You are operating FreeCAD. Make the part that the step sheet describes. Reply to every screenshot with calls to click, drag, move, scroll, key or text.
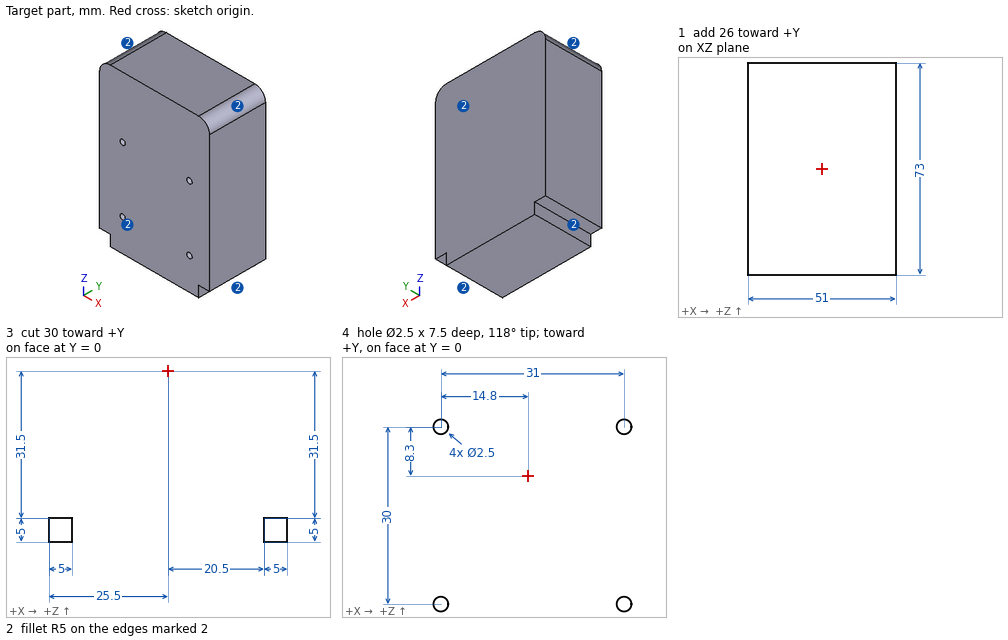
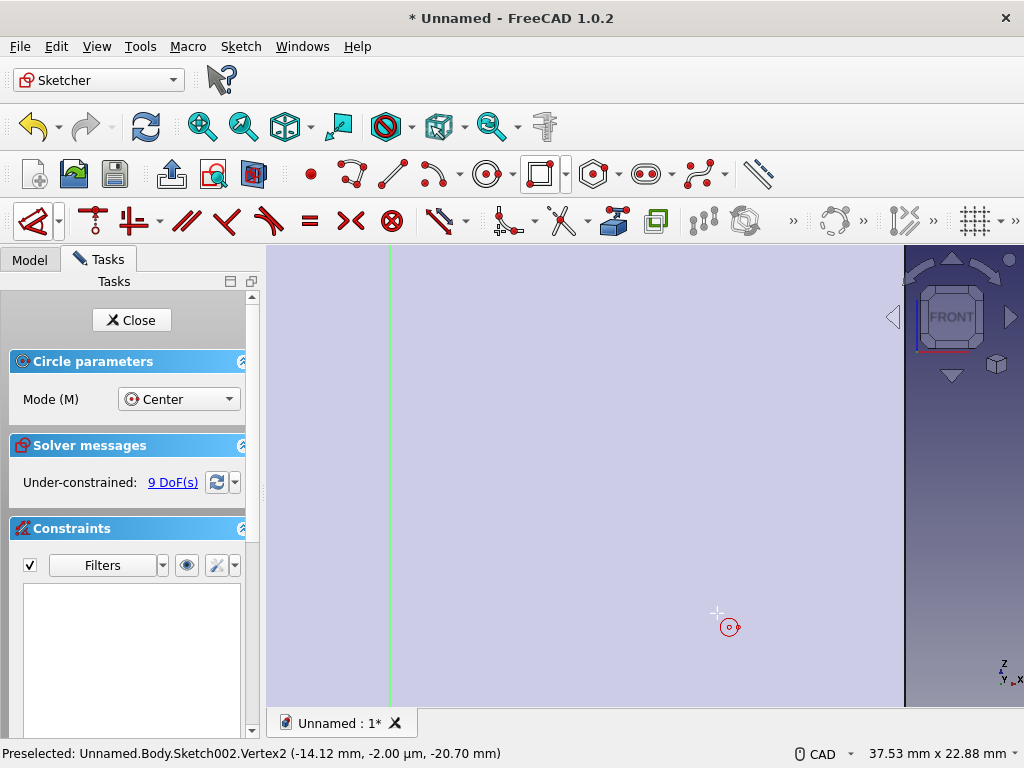
click(717, 611)
click(735, 593)
key(Escape)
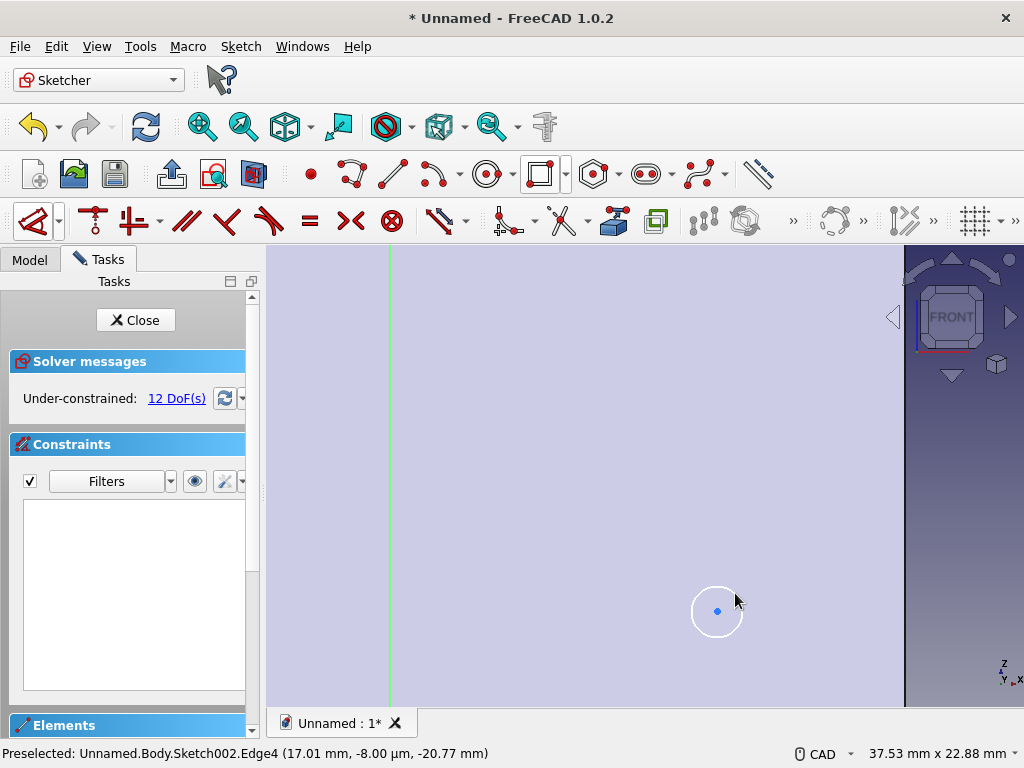
scroll(717, 613, down, 4)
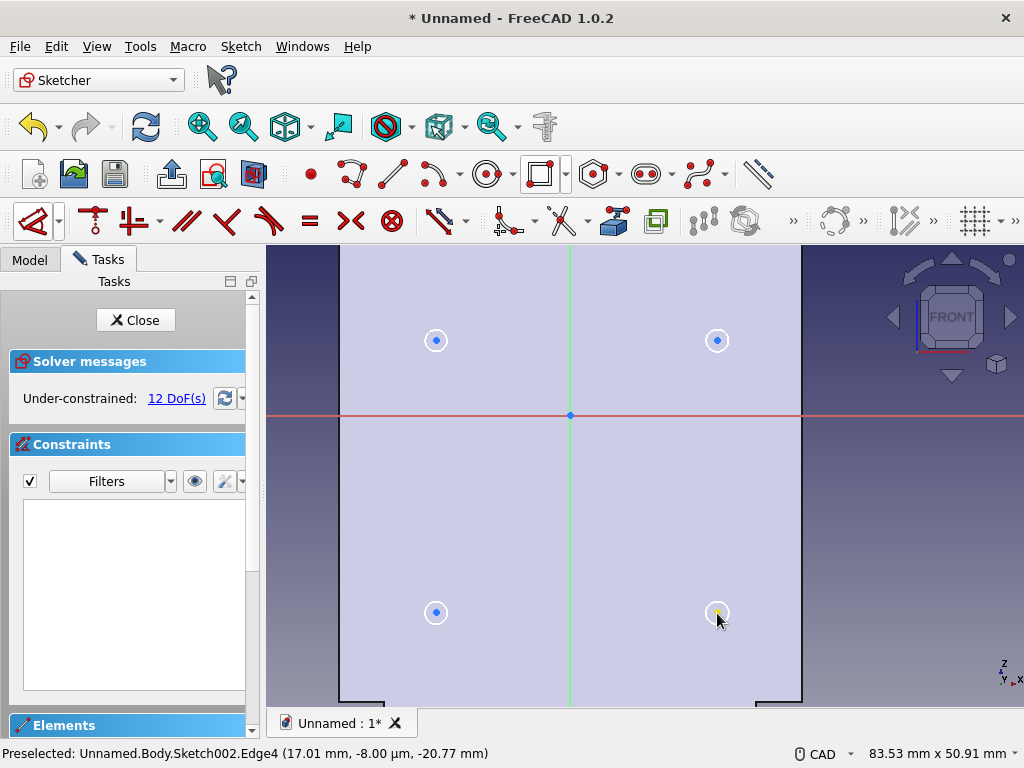
scroll(444, 333, up, 2)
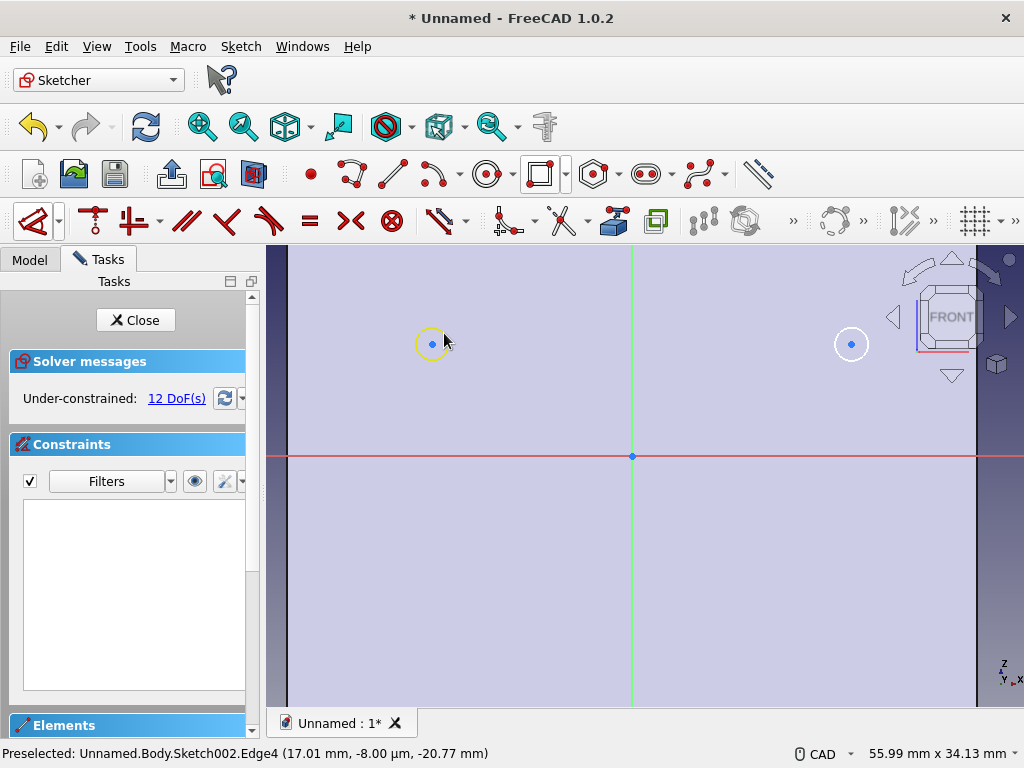
click(443, 333)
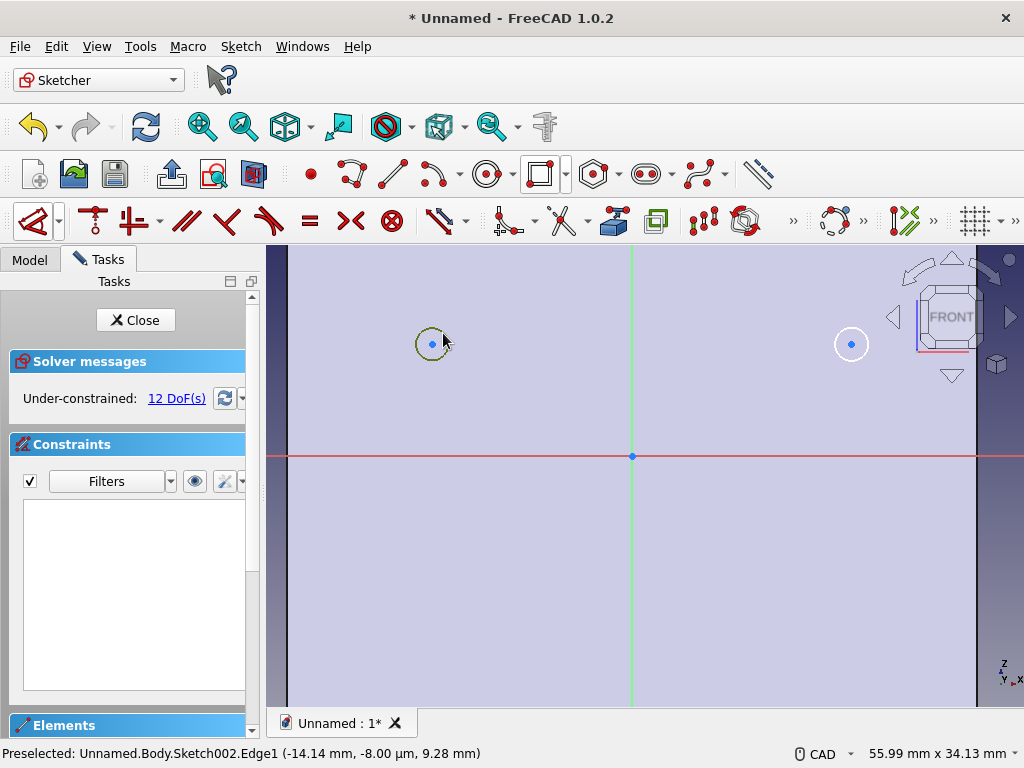
click(840, 333)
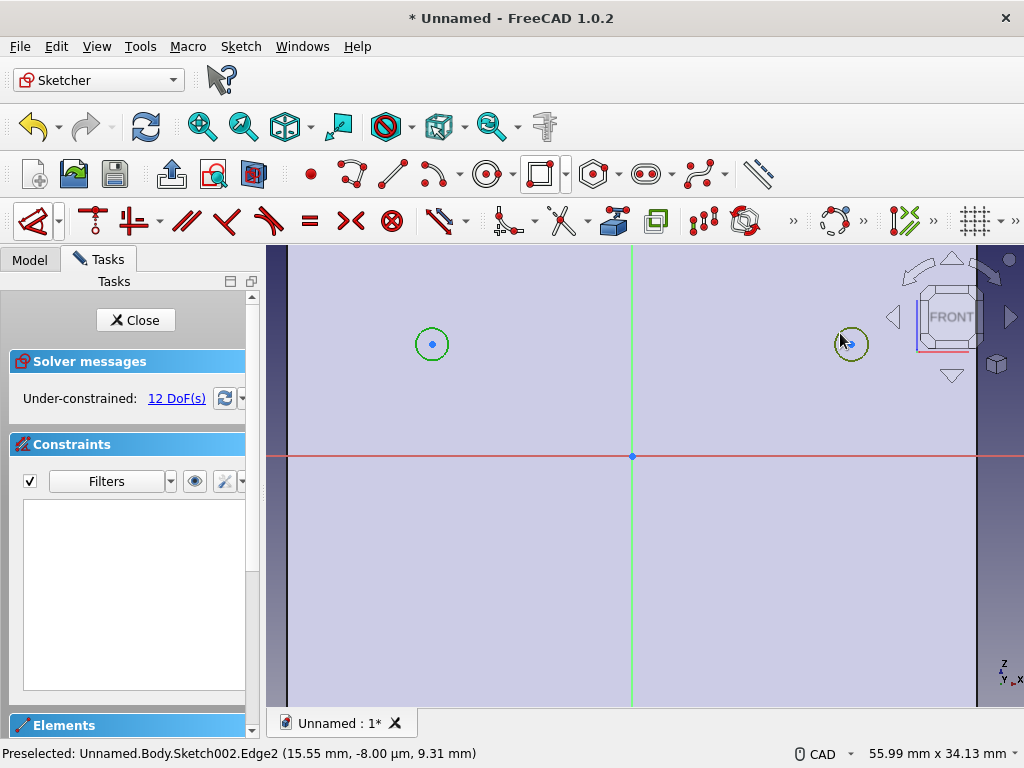
scroll(444, 332, down, 2)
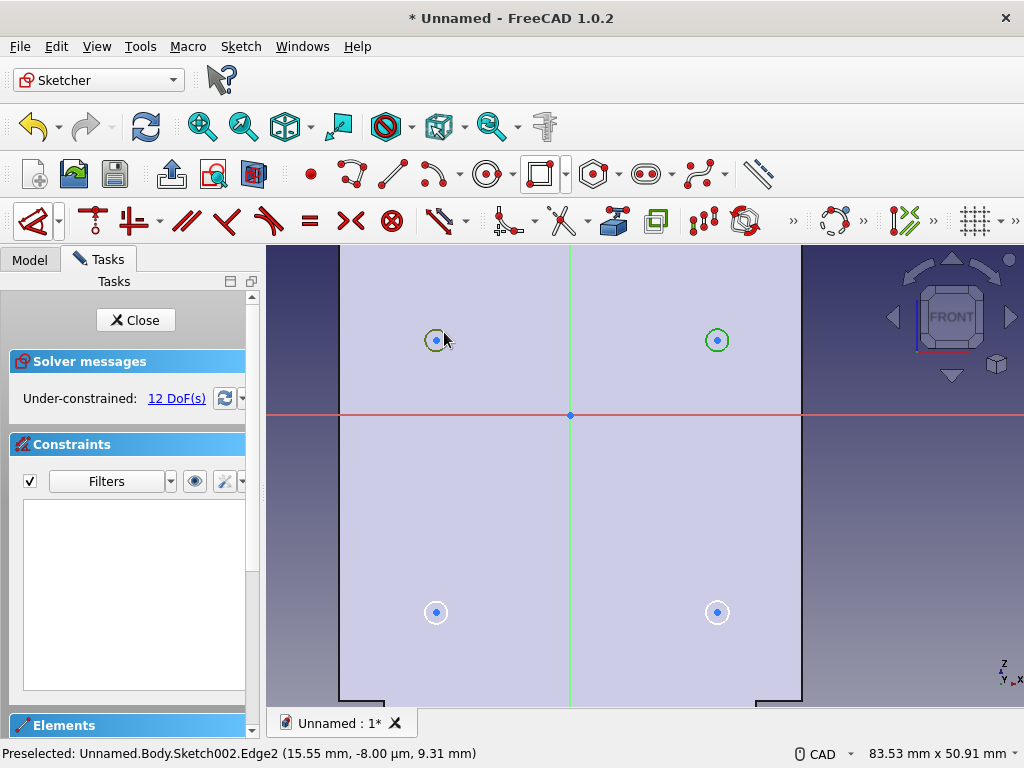
scroll(444, 605, up, 2)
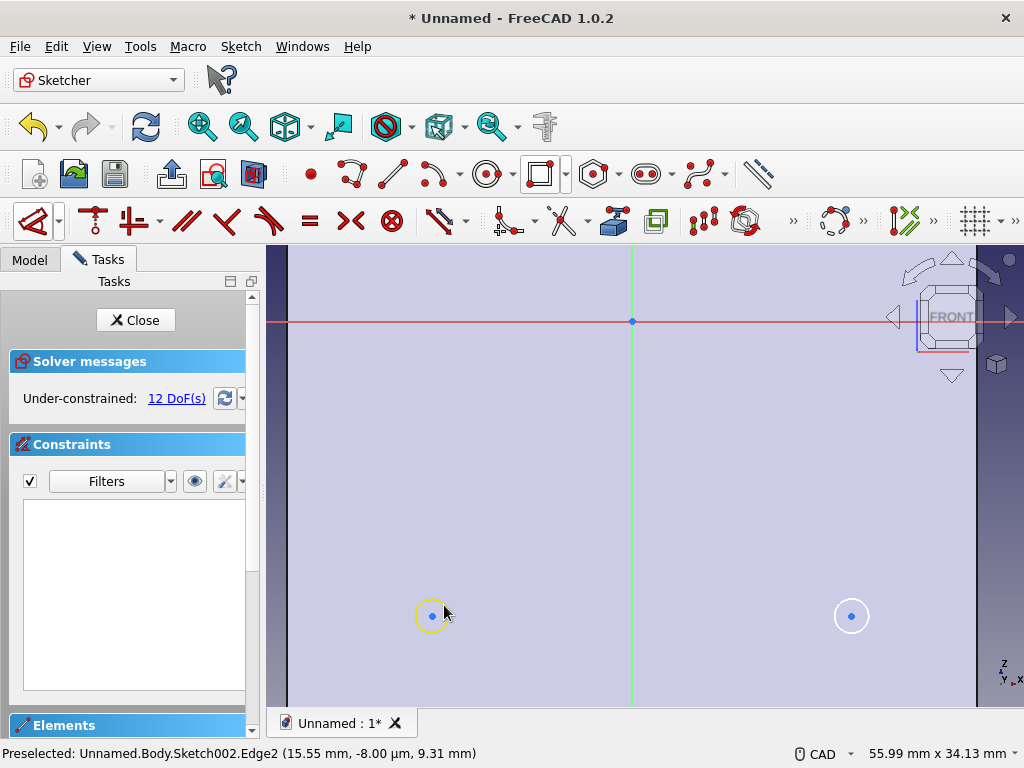
click(444, 604)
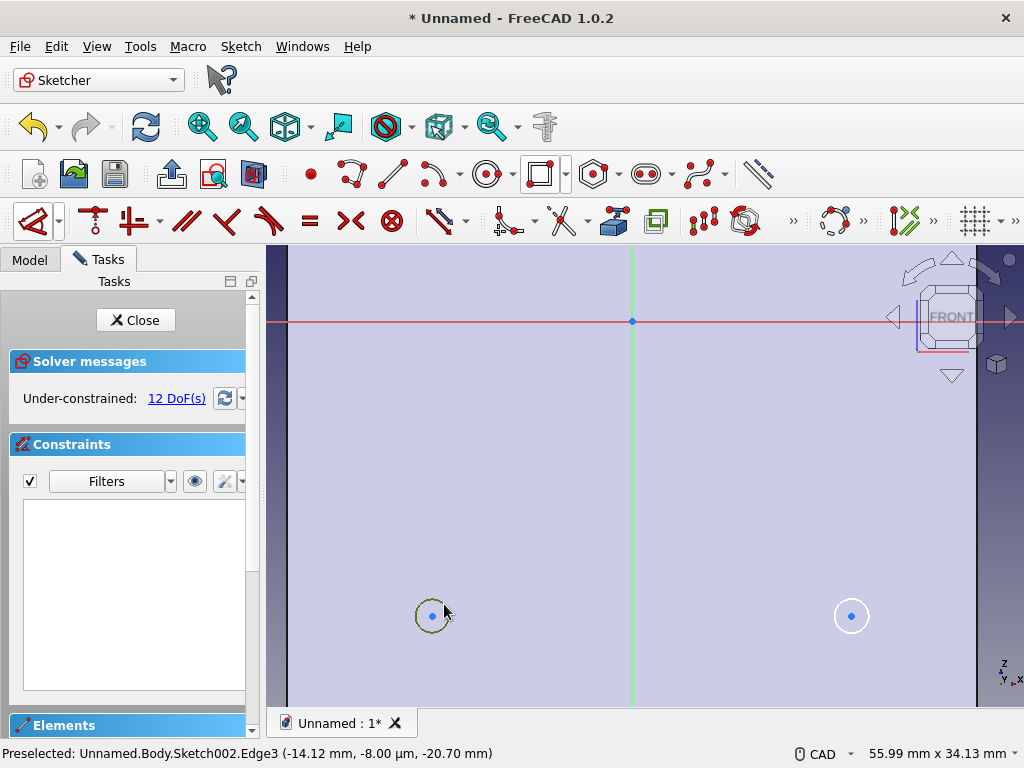
click(840, 604)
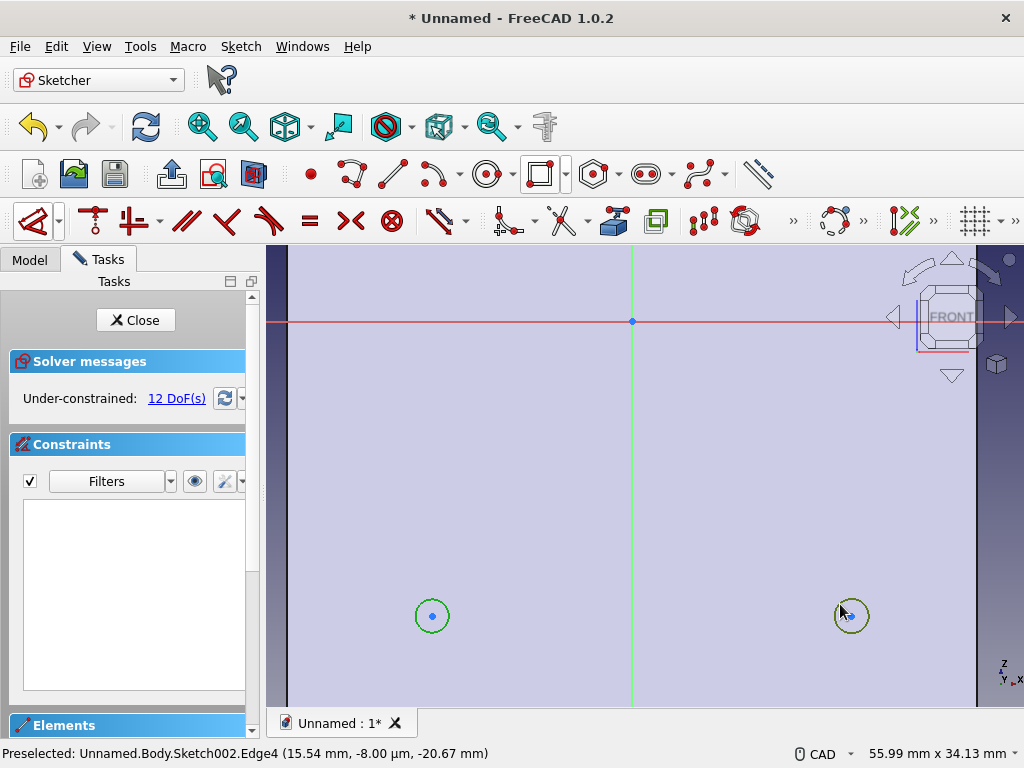
key(e)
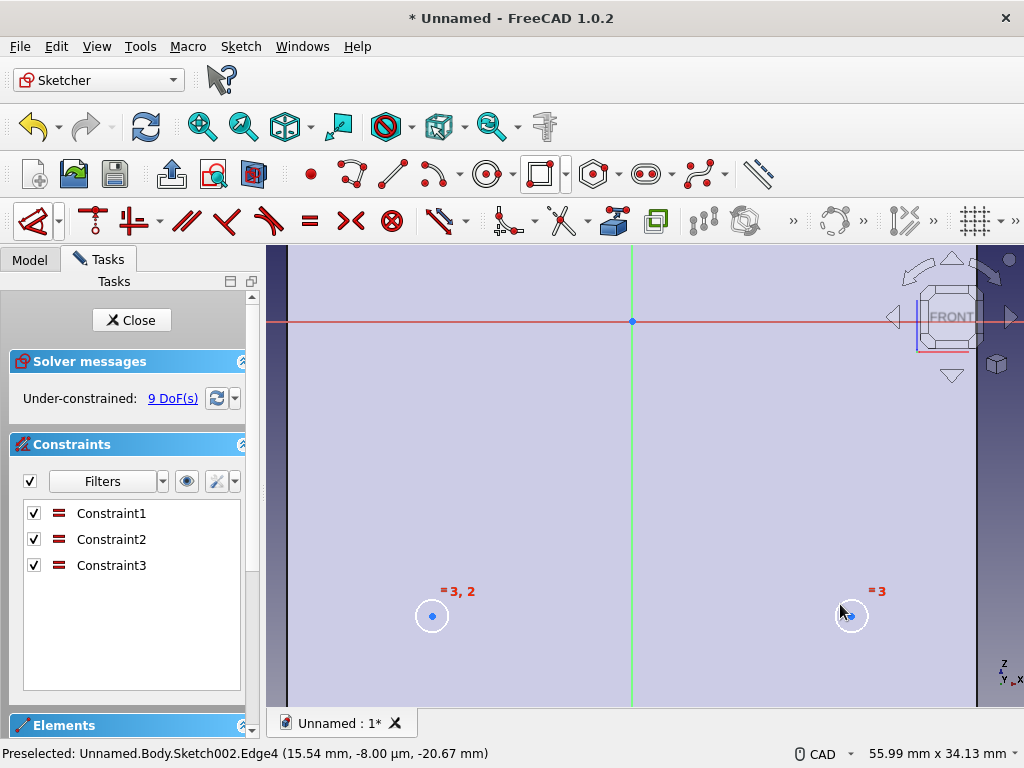
scroll(444, 605, down, 2)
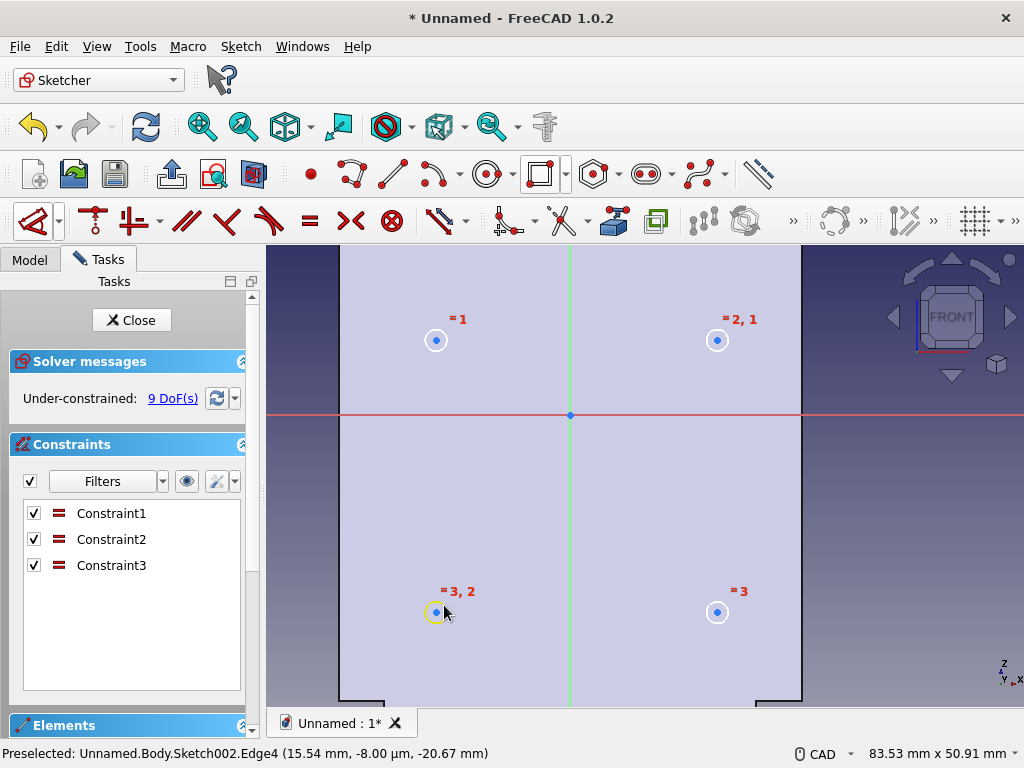
click(436, 340)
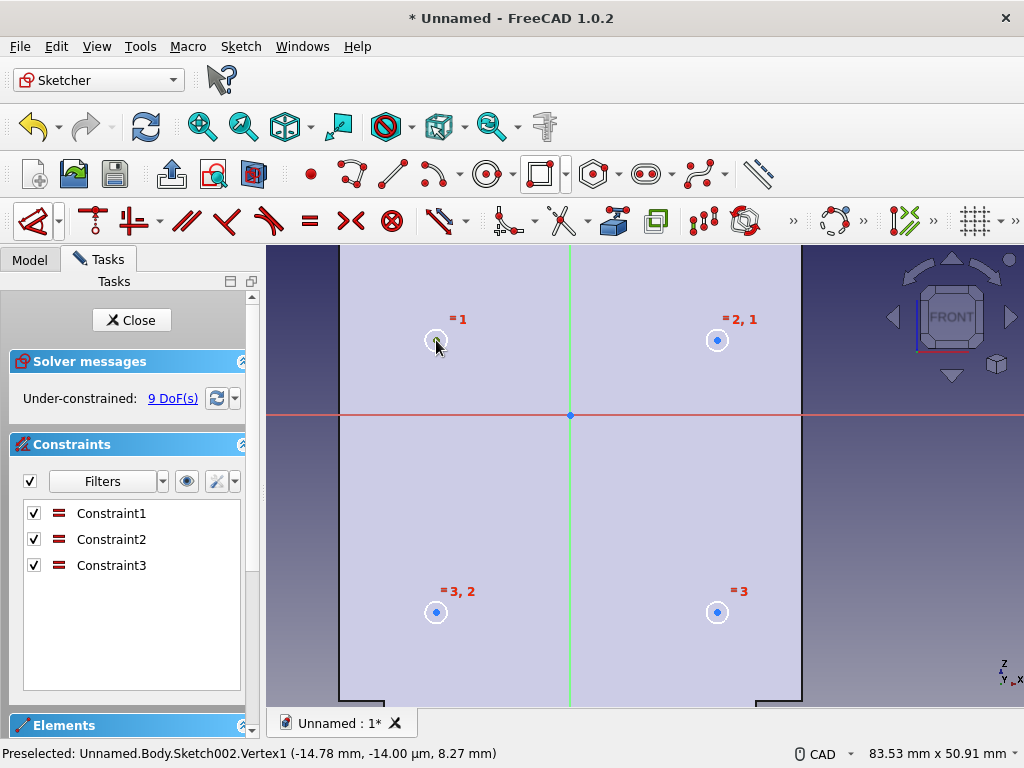
click(717, 340)